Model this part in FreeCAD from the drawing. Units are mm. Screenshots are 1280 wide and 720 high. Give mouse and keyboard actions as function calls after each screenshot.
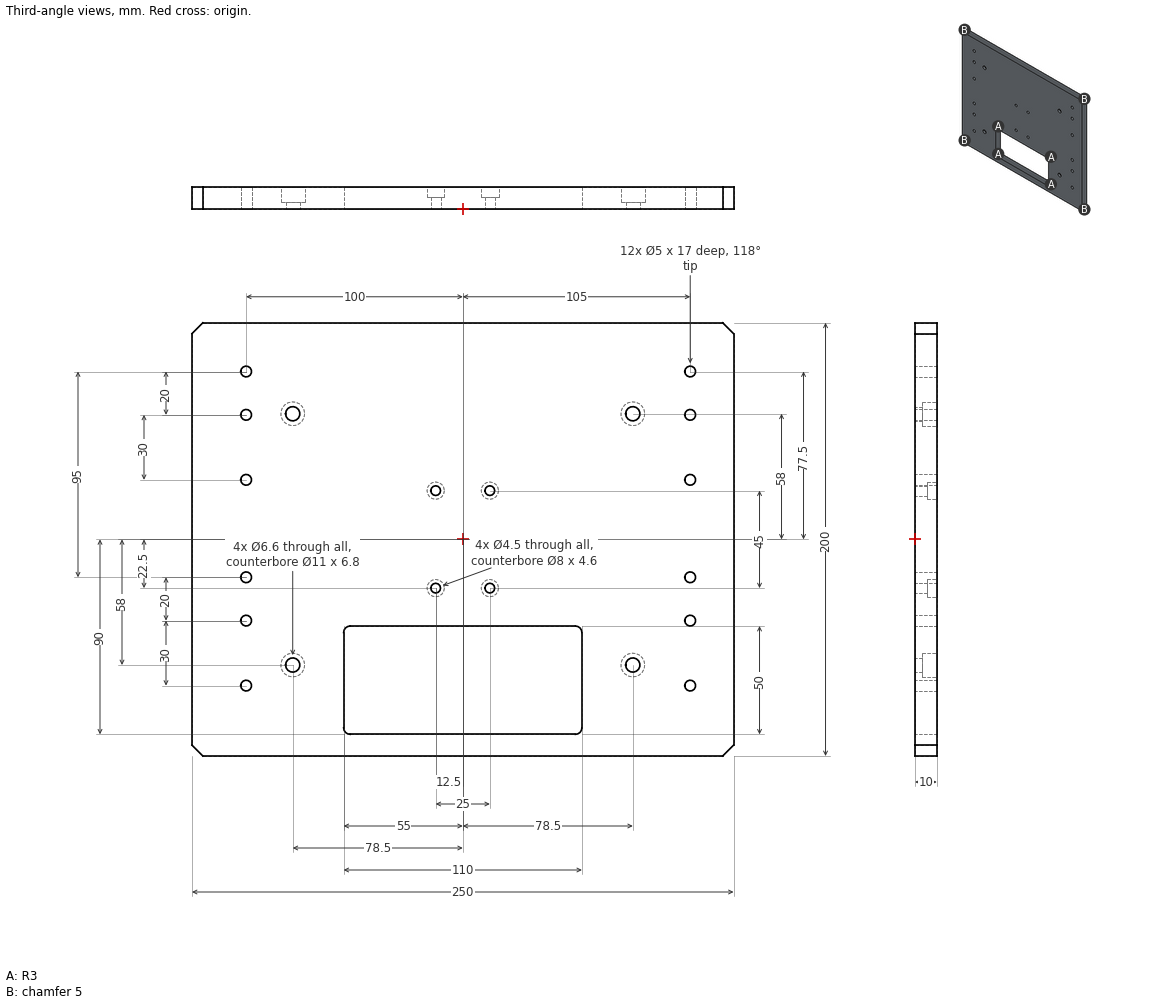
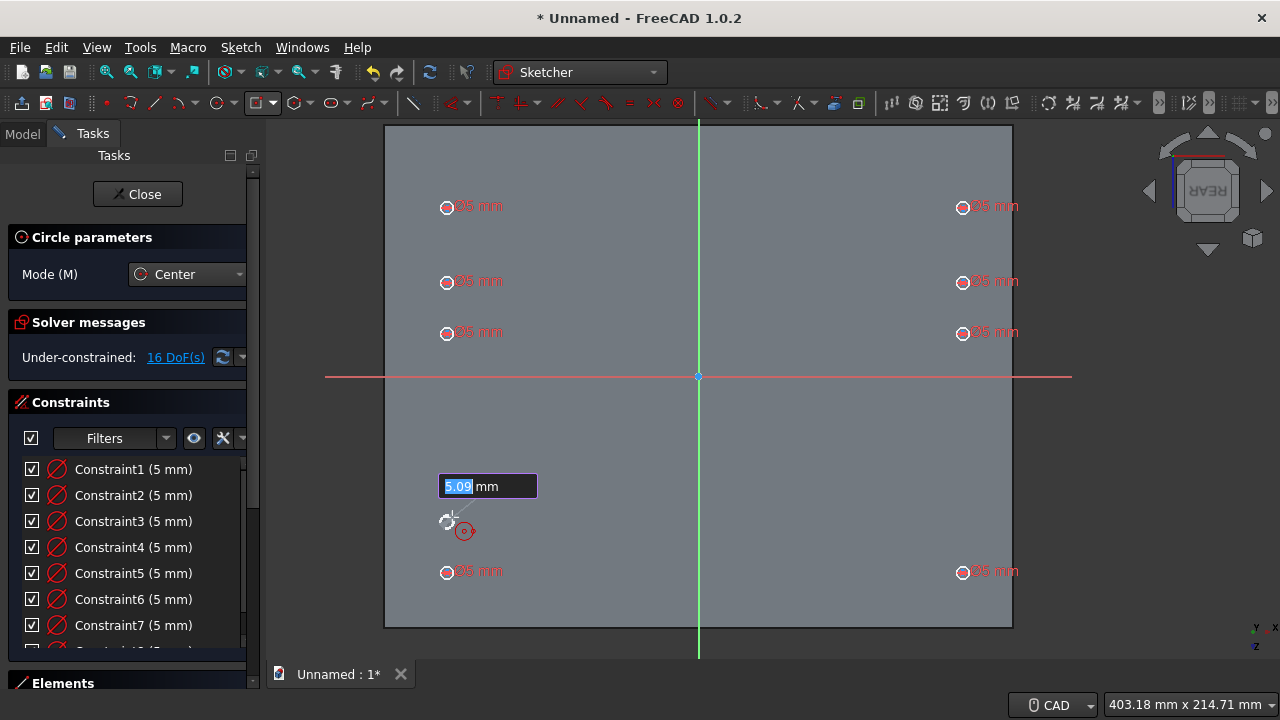
text(5)
key(Return)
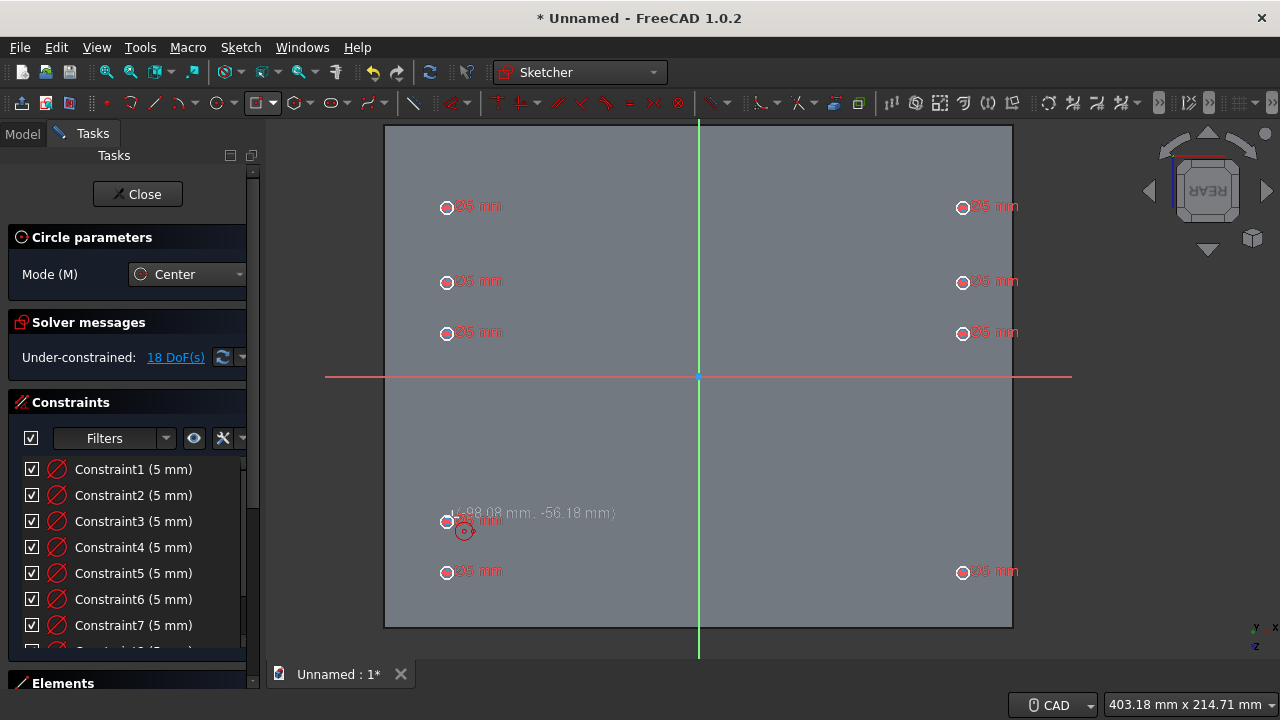
scroll(447, 446, up, 7)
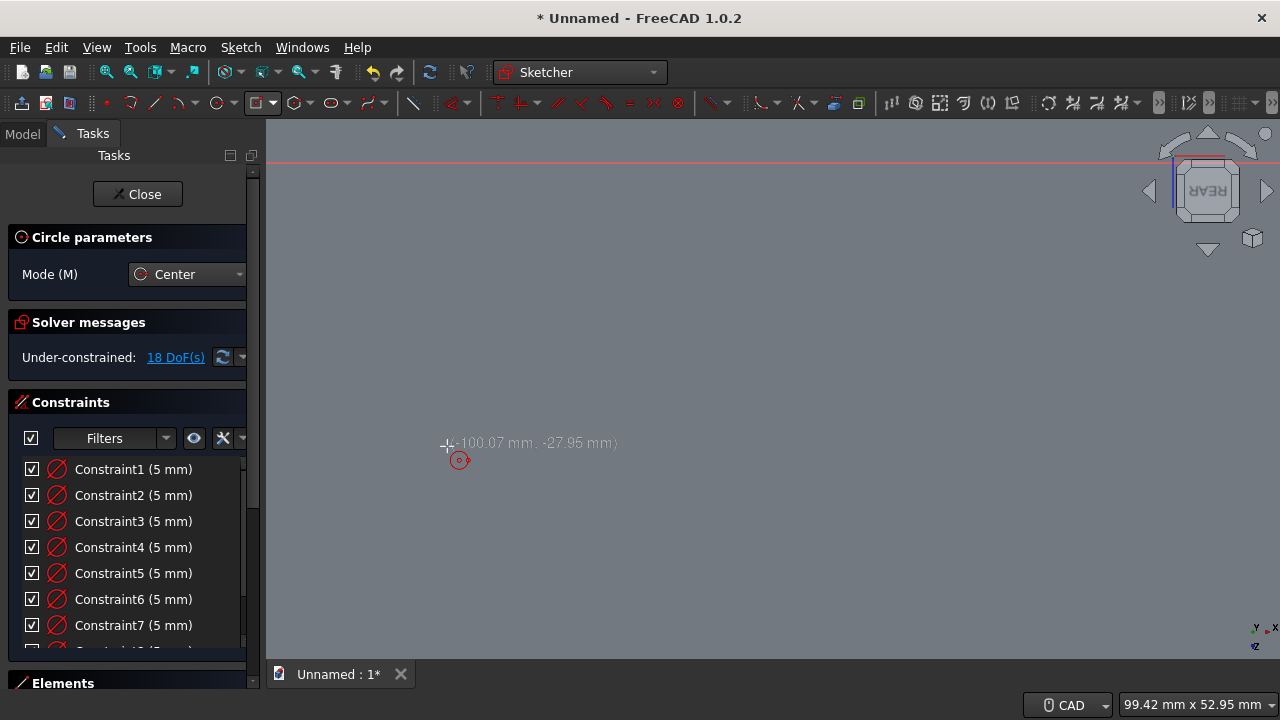
scroll(447, 446, down, 7)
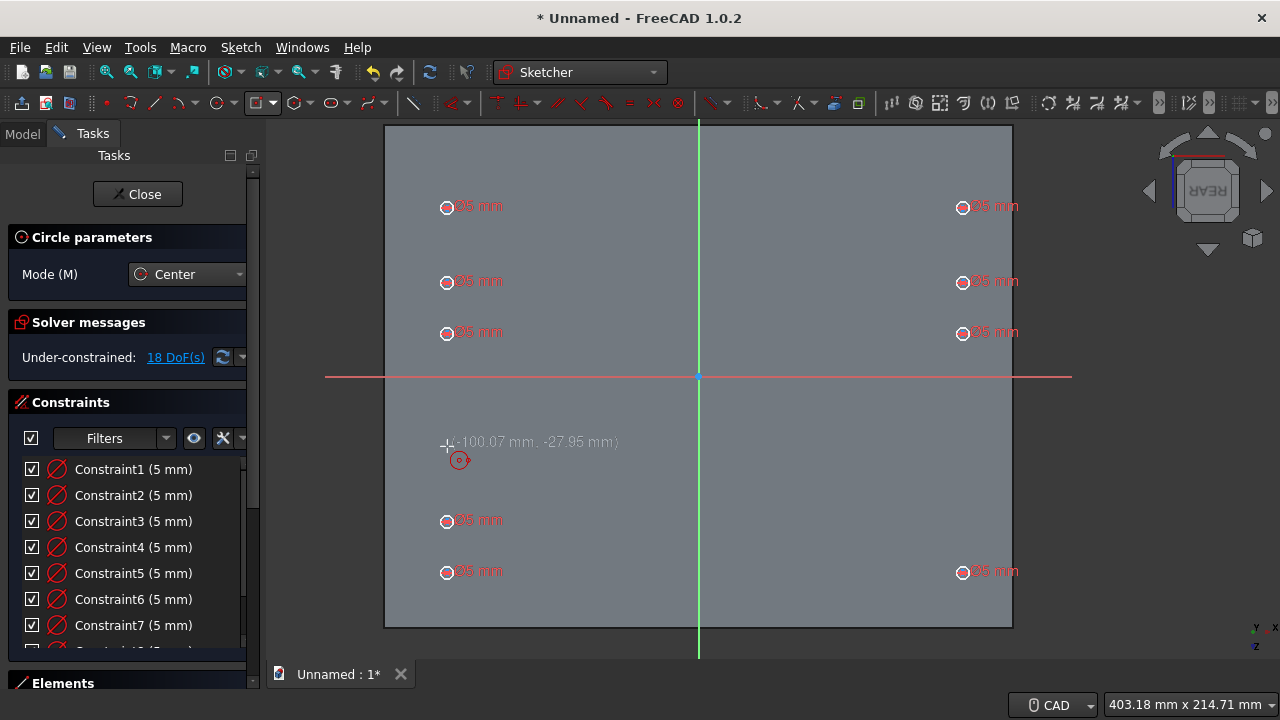
click(447, 446)
move(452, 441)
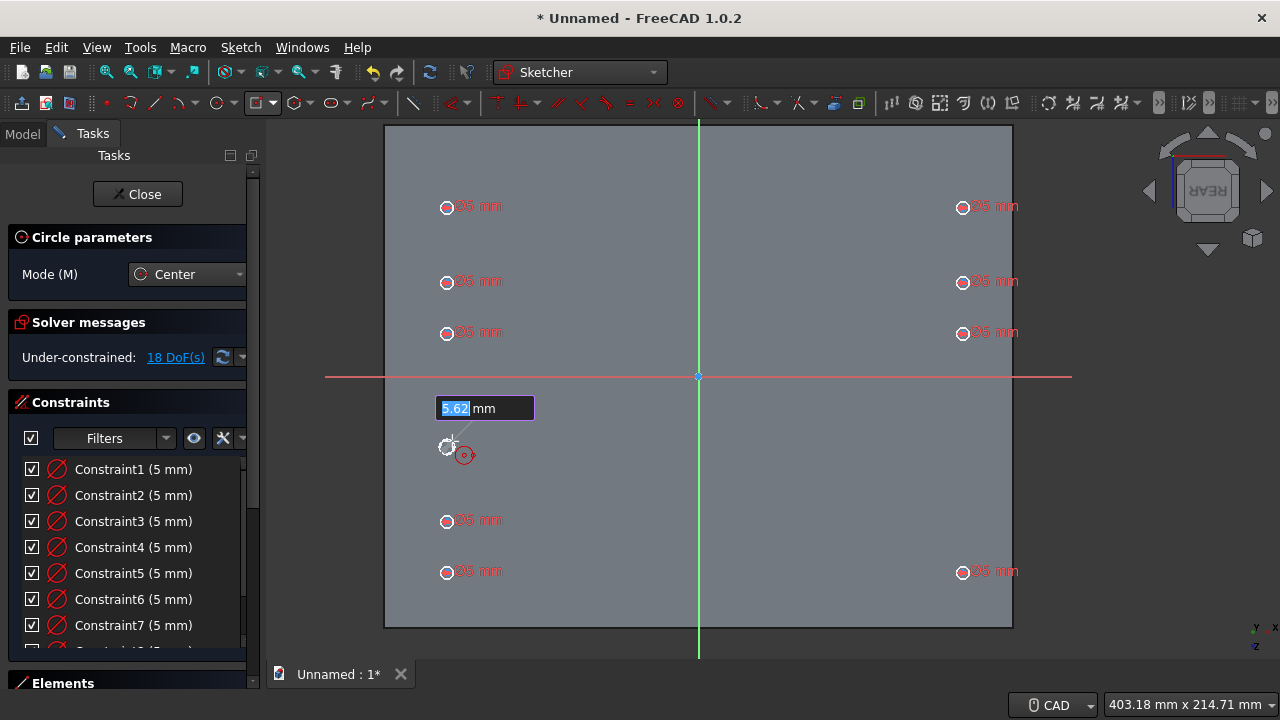
text(5)
key(Return)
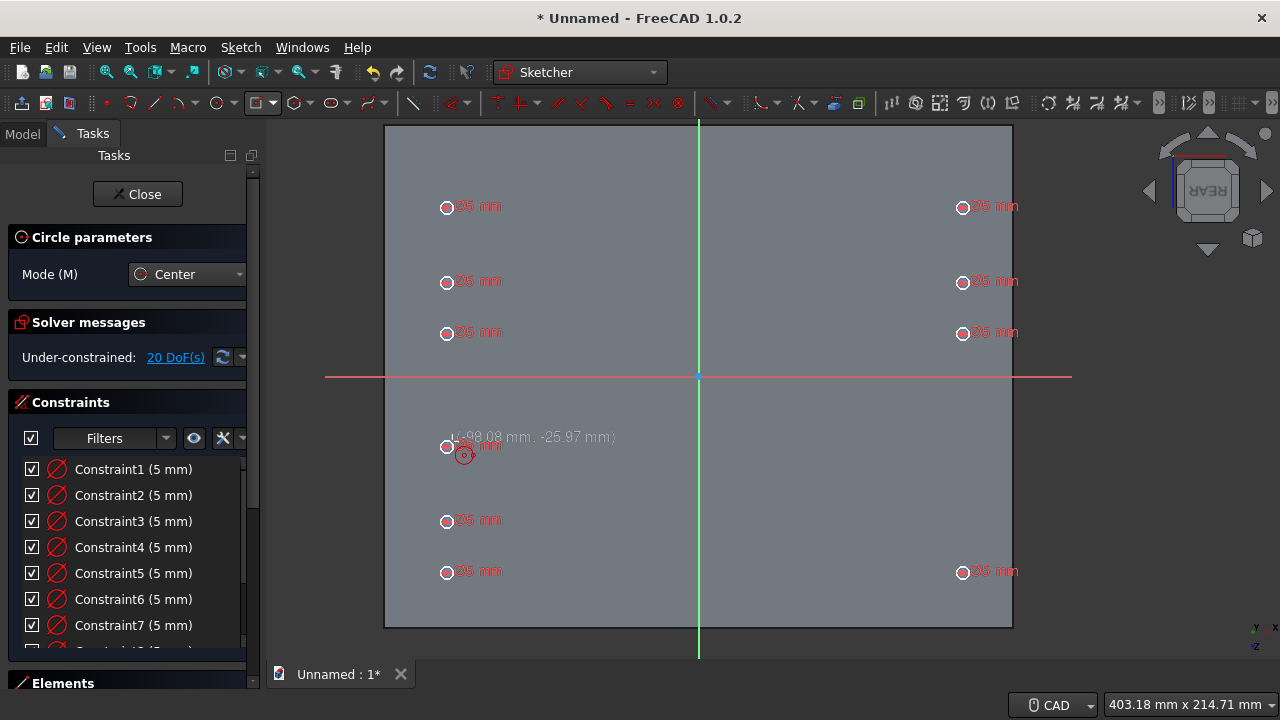
scroll(963, 521, up, 7)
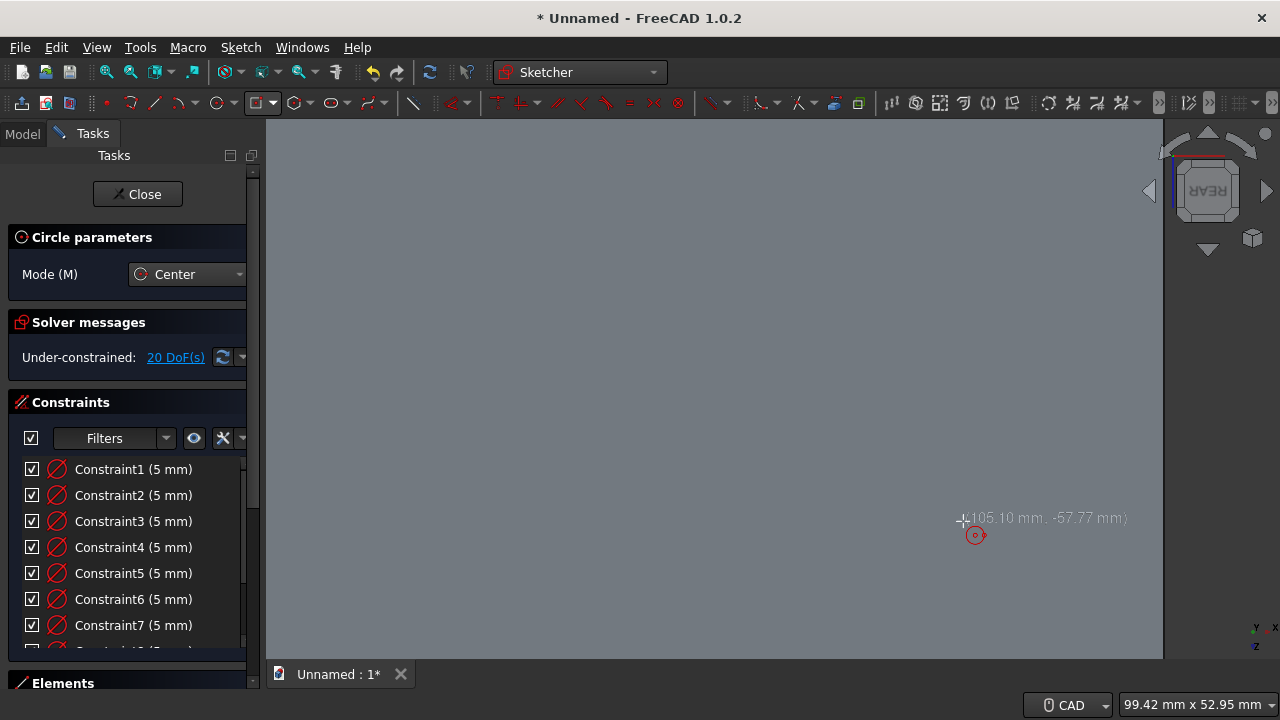
scroll(963, 521, down, 7)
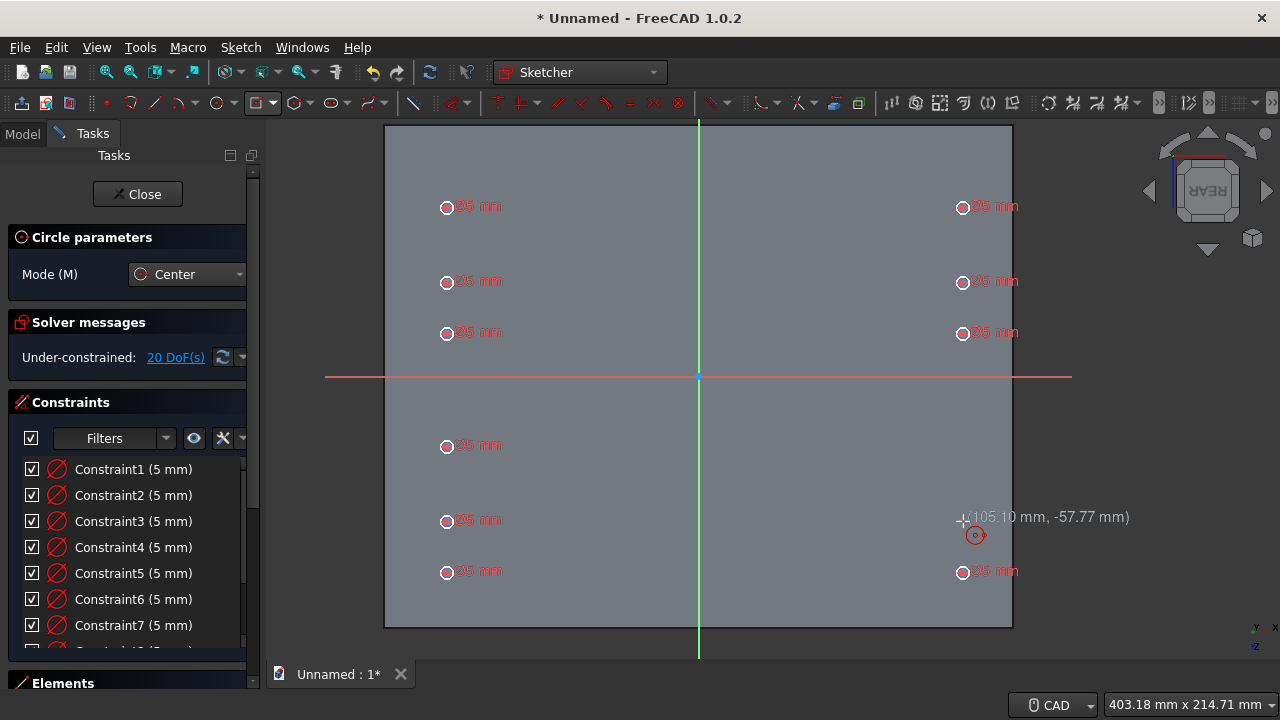
click(963, 521)
move(967, 517)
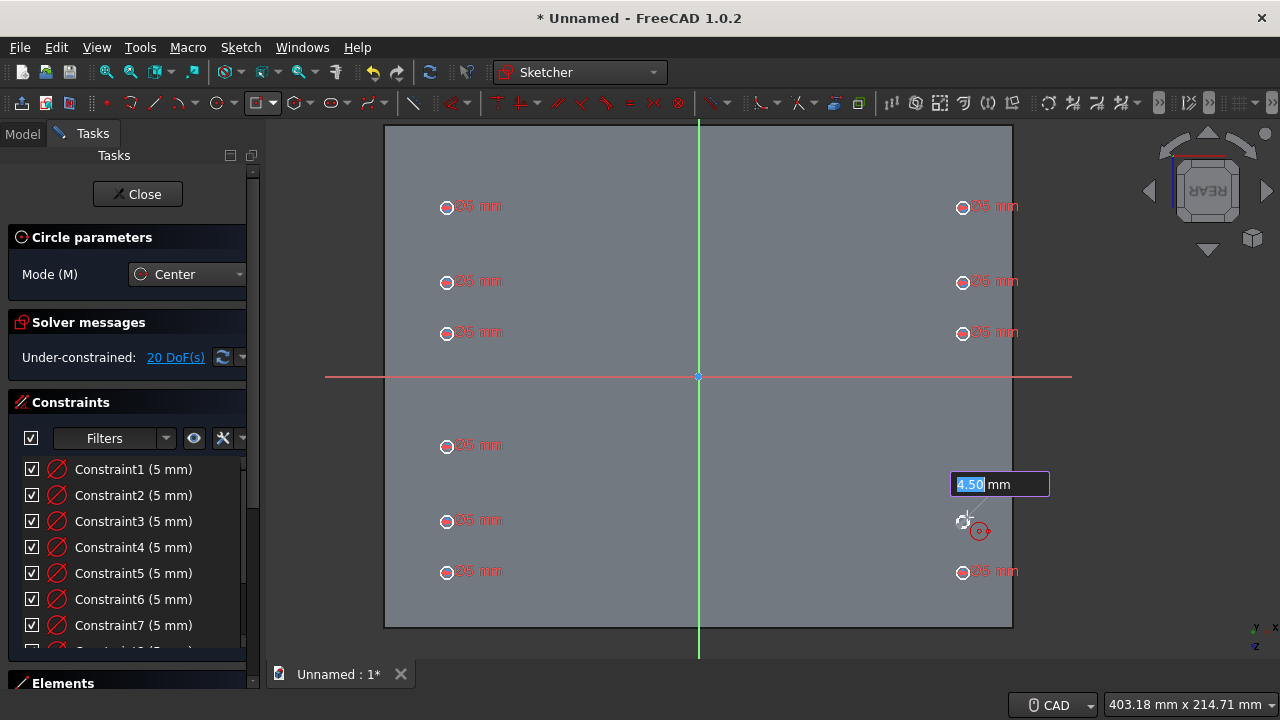
text(5)
key(Return)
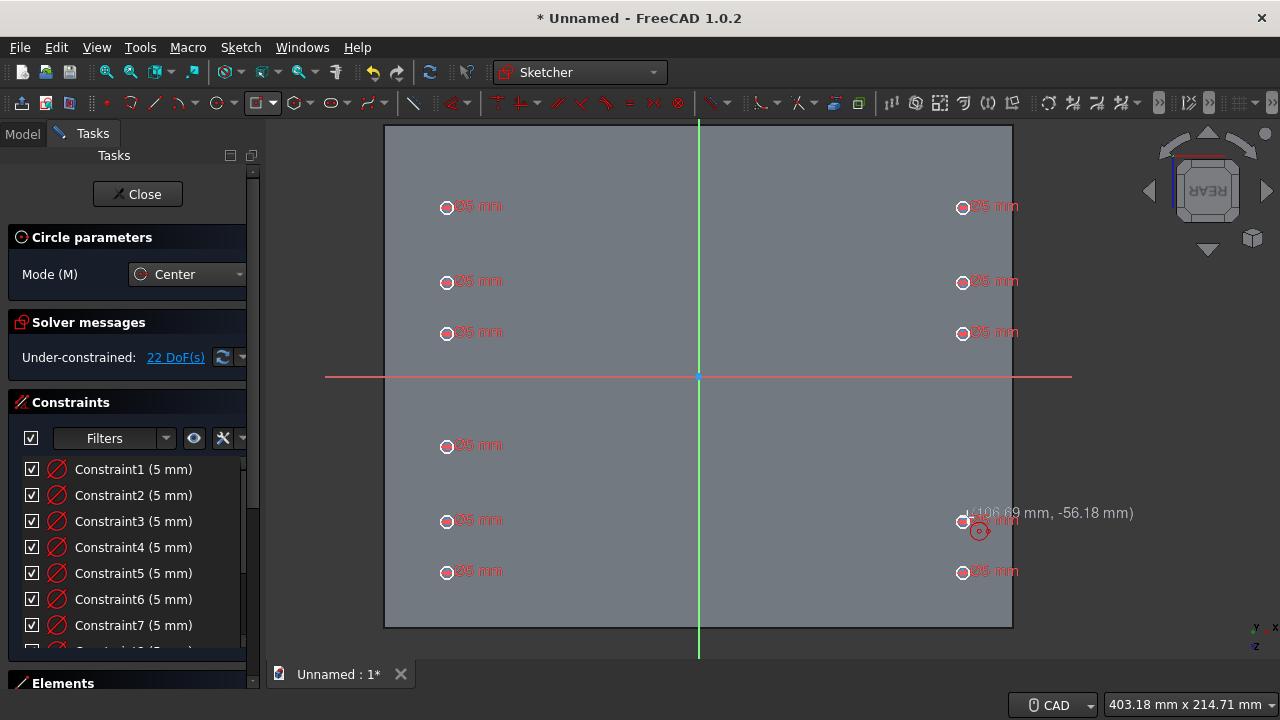
scroll(963, 446, up, 7)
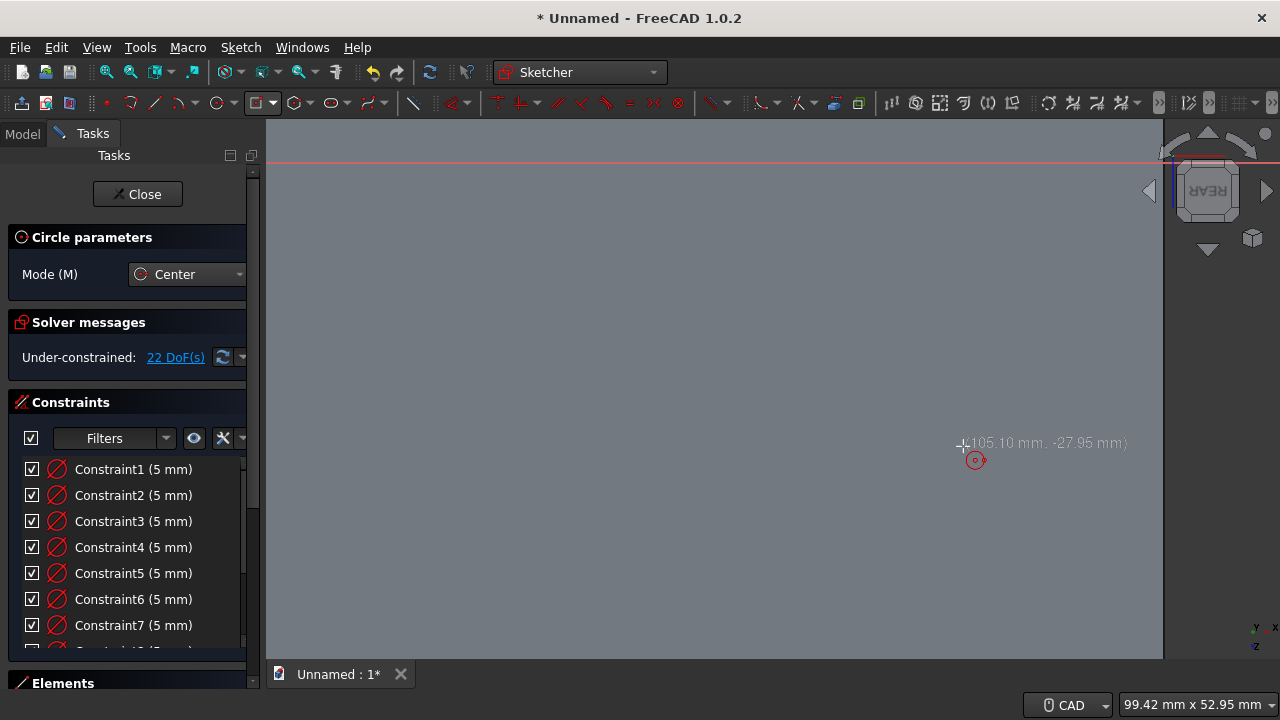
scroll(963, 446, down, 7)